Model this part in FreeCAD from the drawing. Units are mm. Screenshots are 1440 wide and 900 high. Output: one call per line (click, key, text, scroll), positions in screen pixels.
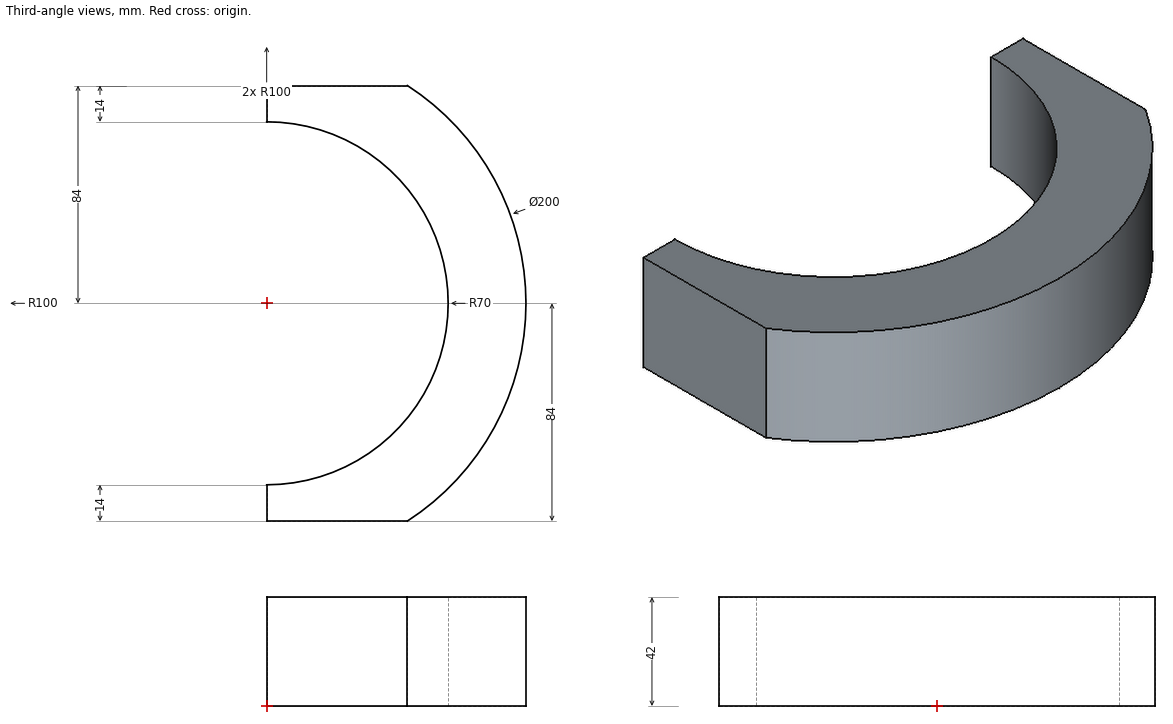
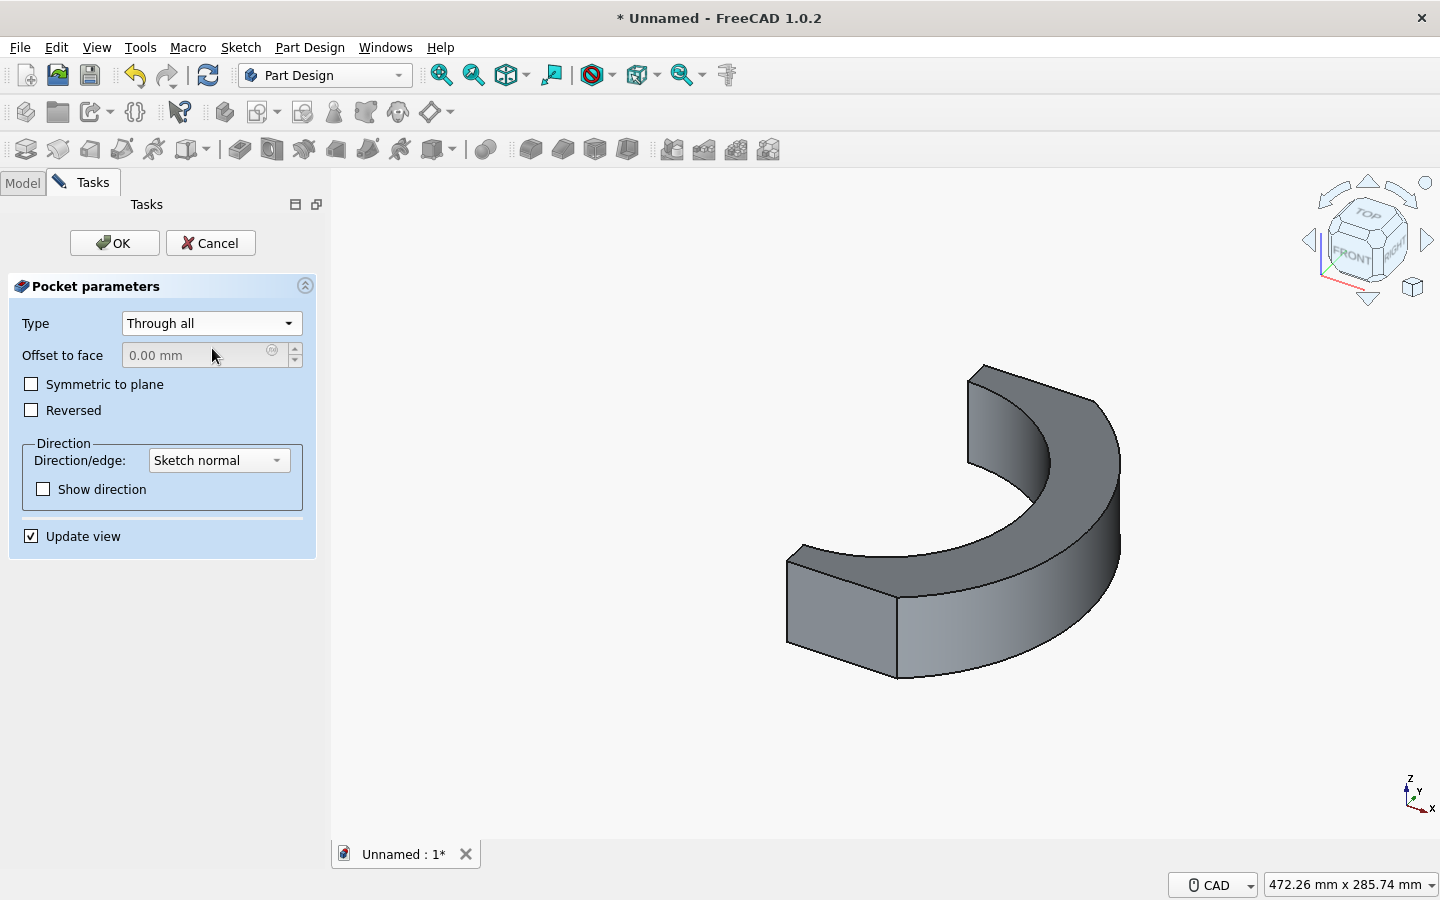
click(115, 243)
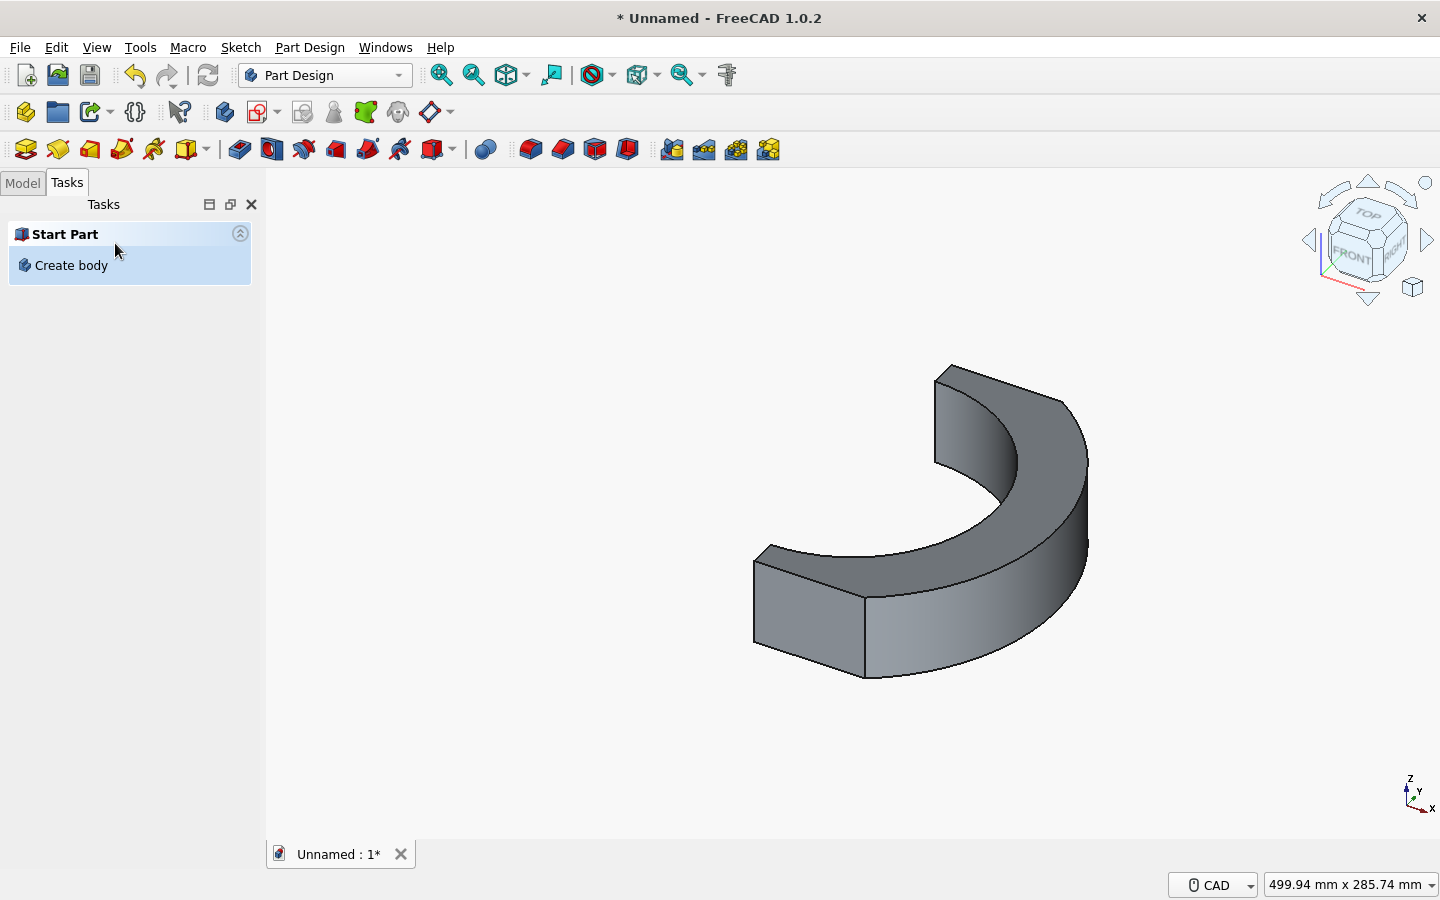
key(0)